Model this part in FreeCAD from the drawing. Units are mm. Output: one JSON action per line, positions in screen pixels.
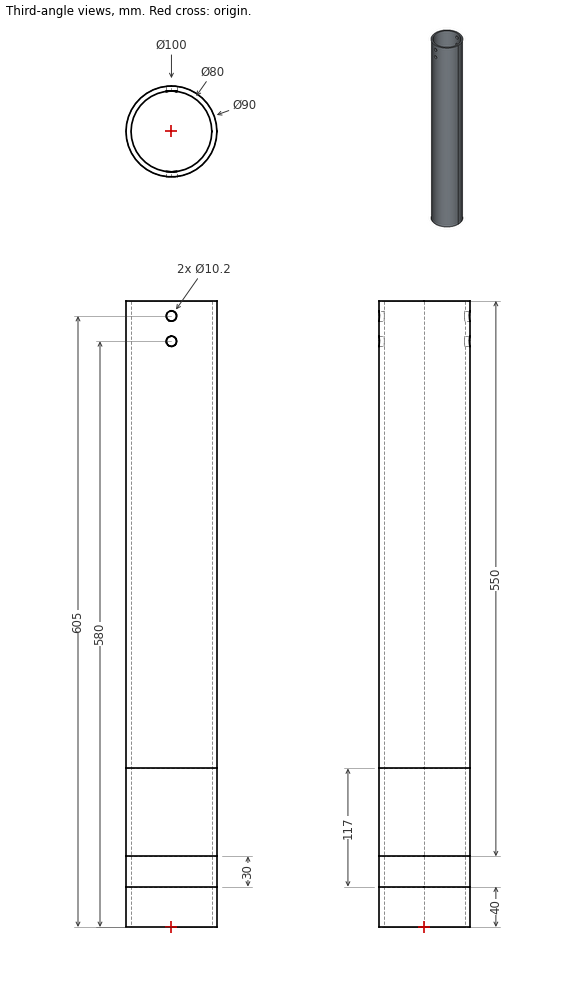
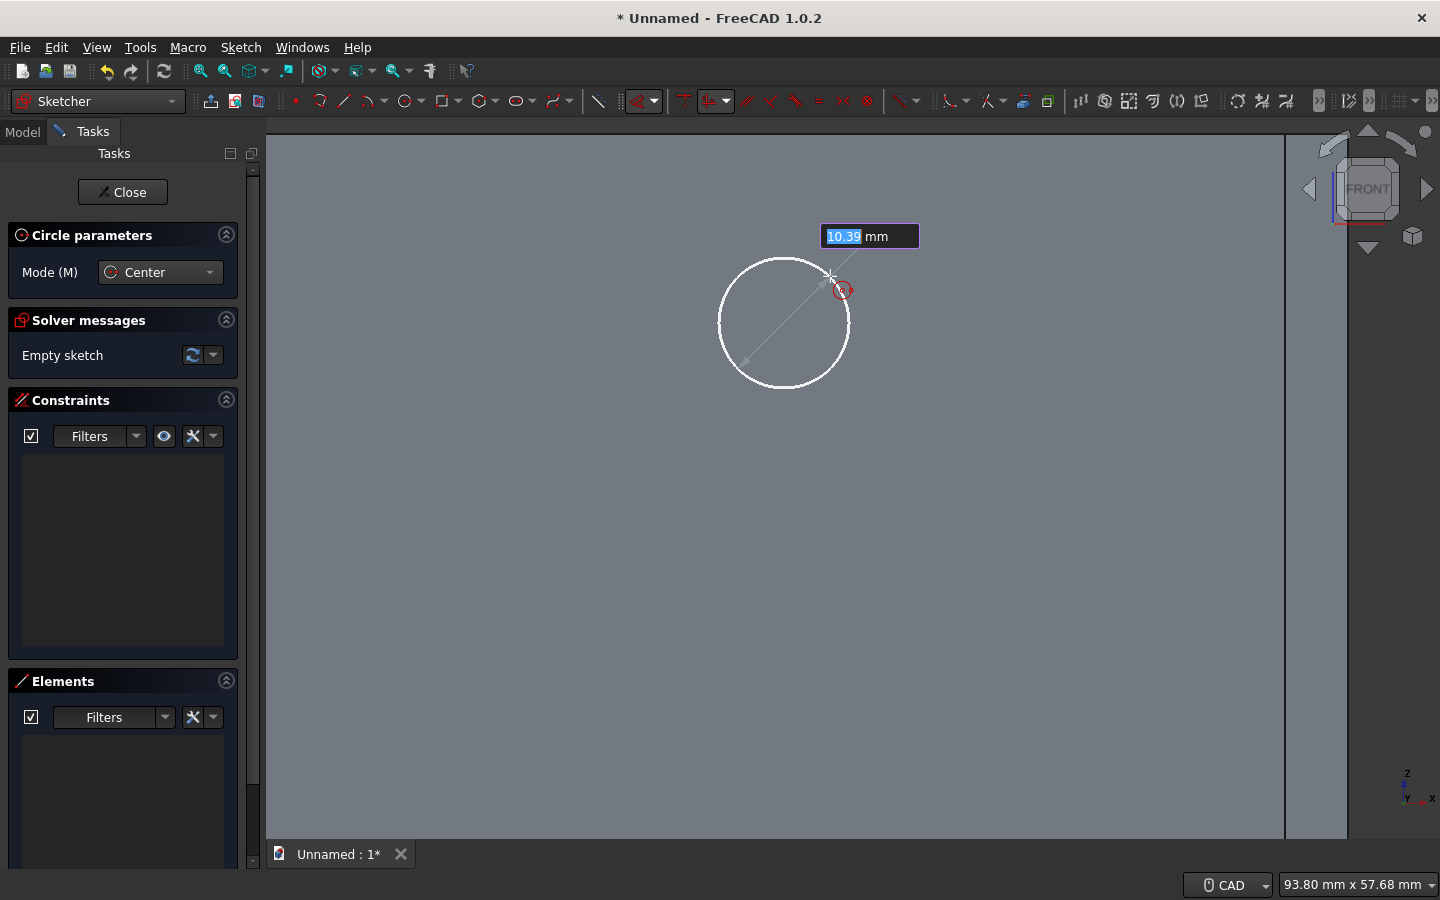
{"action": "type", "text": "10.2"}
{"action": "key", "text": "Return"}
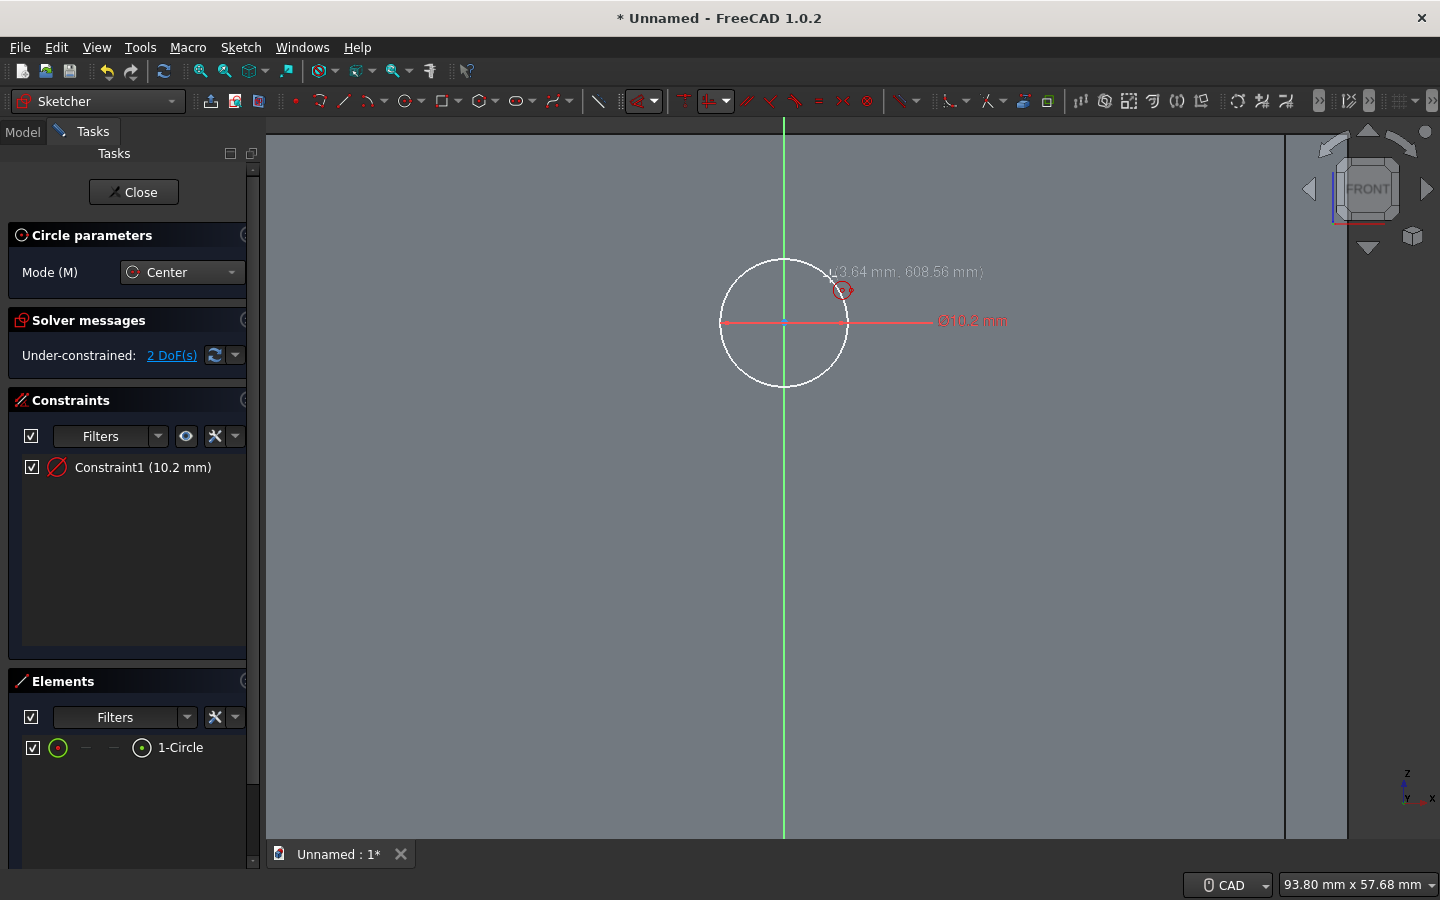
{"action": "left_click", "coordinate": [784, 634]}
{"action": "mouse_move", "coordinate": [830, 589]}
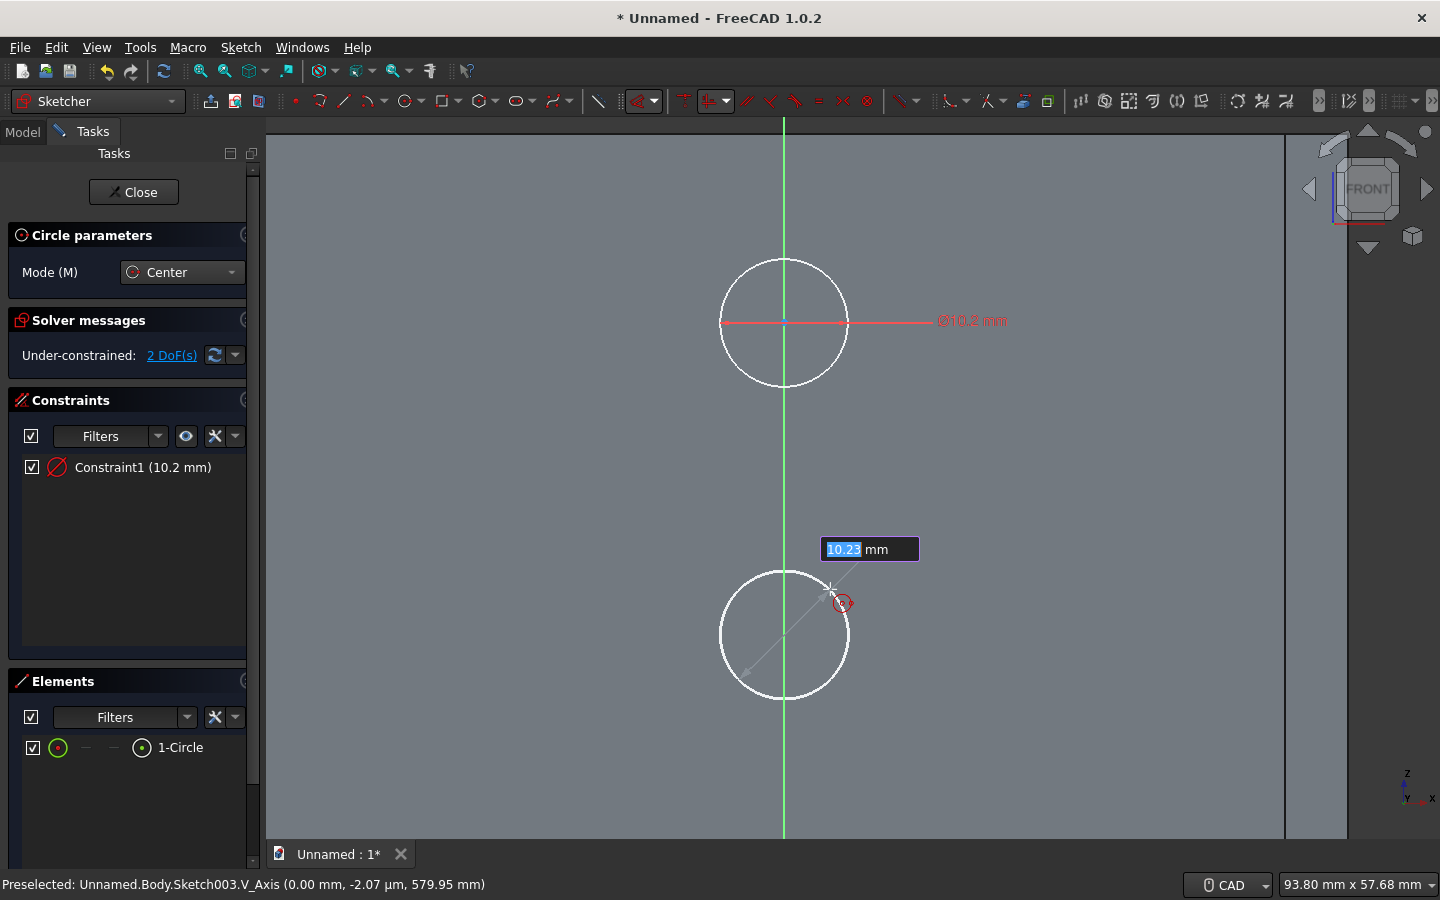
{"action": "type", "text": "10.2"}
{"action": "key", "text": "Return"}
{"action": "key", "text": "Escape"}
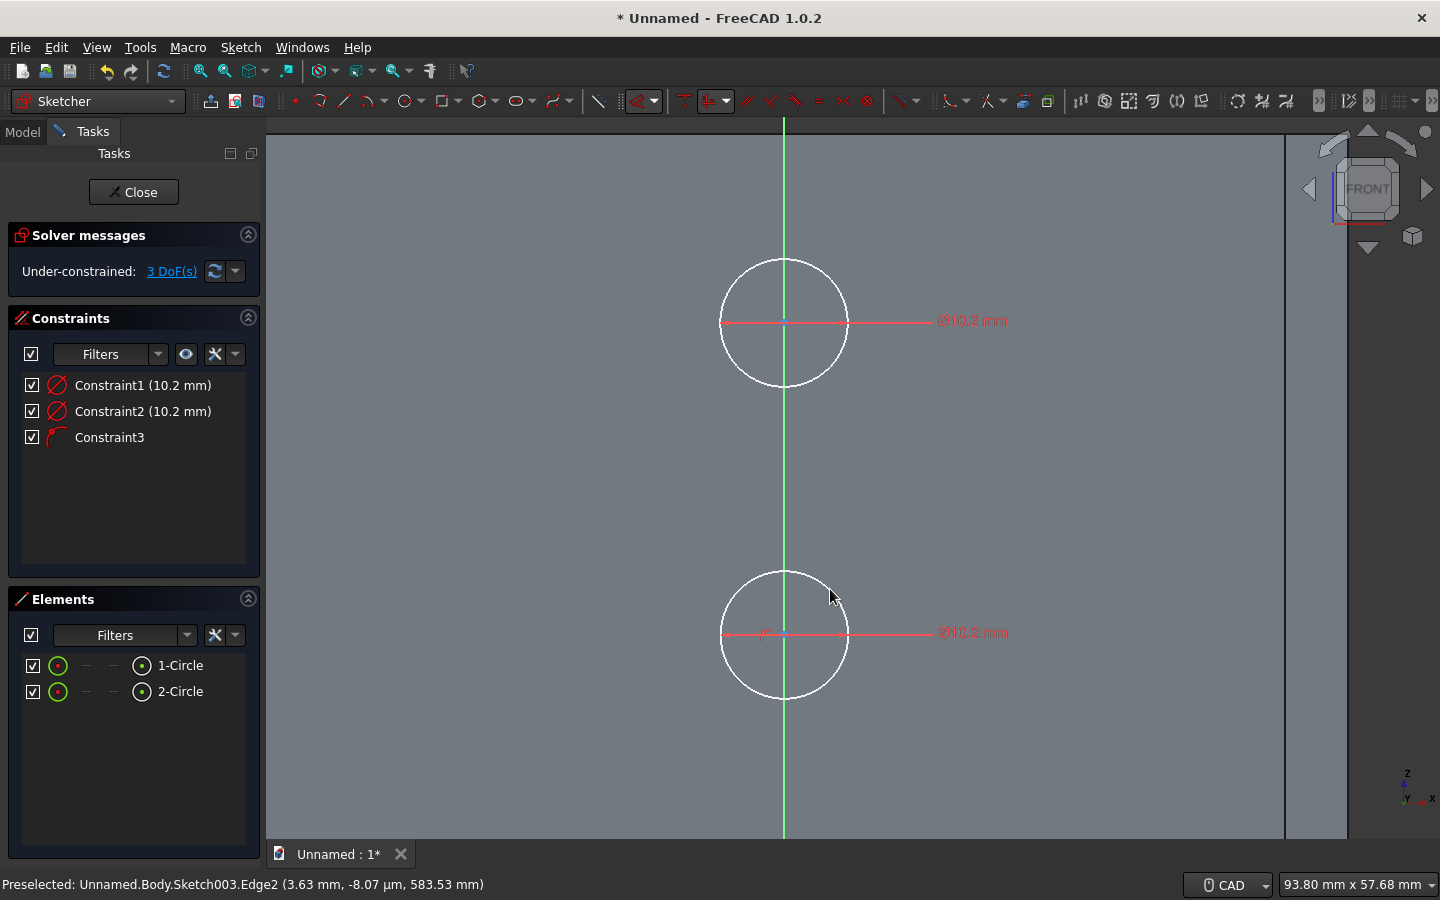
{"action": "left_click", "coordinate": [784, 323]}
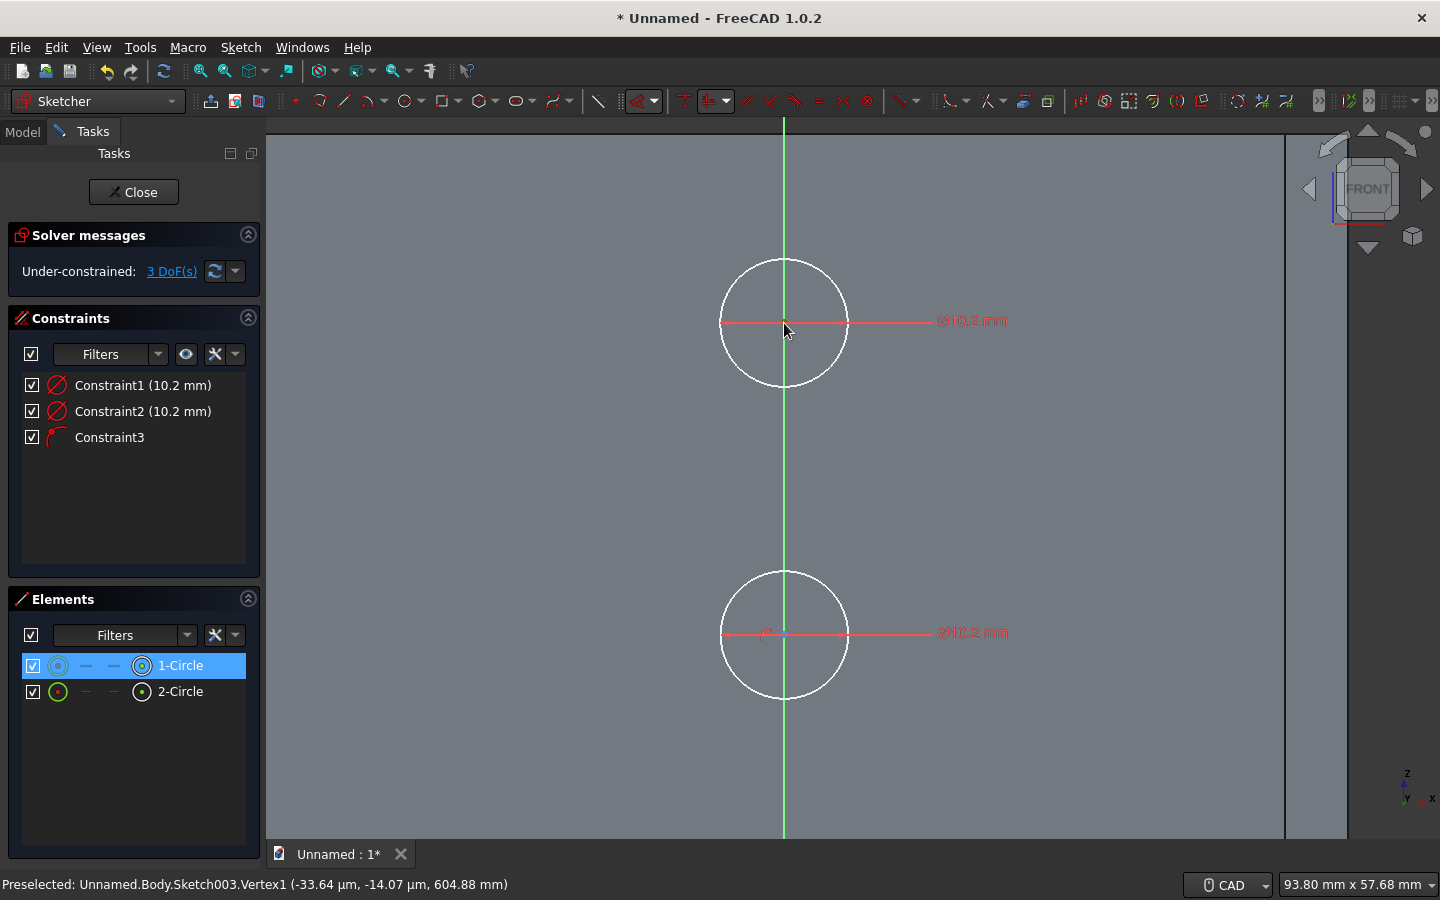
{"action": "left_click", "coordinate": [784, 763]}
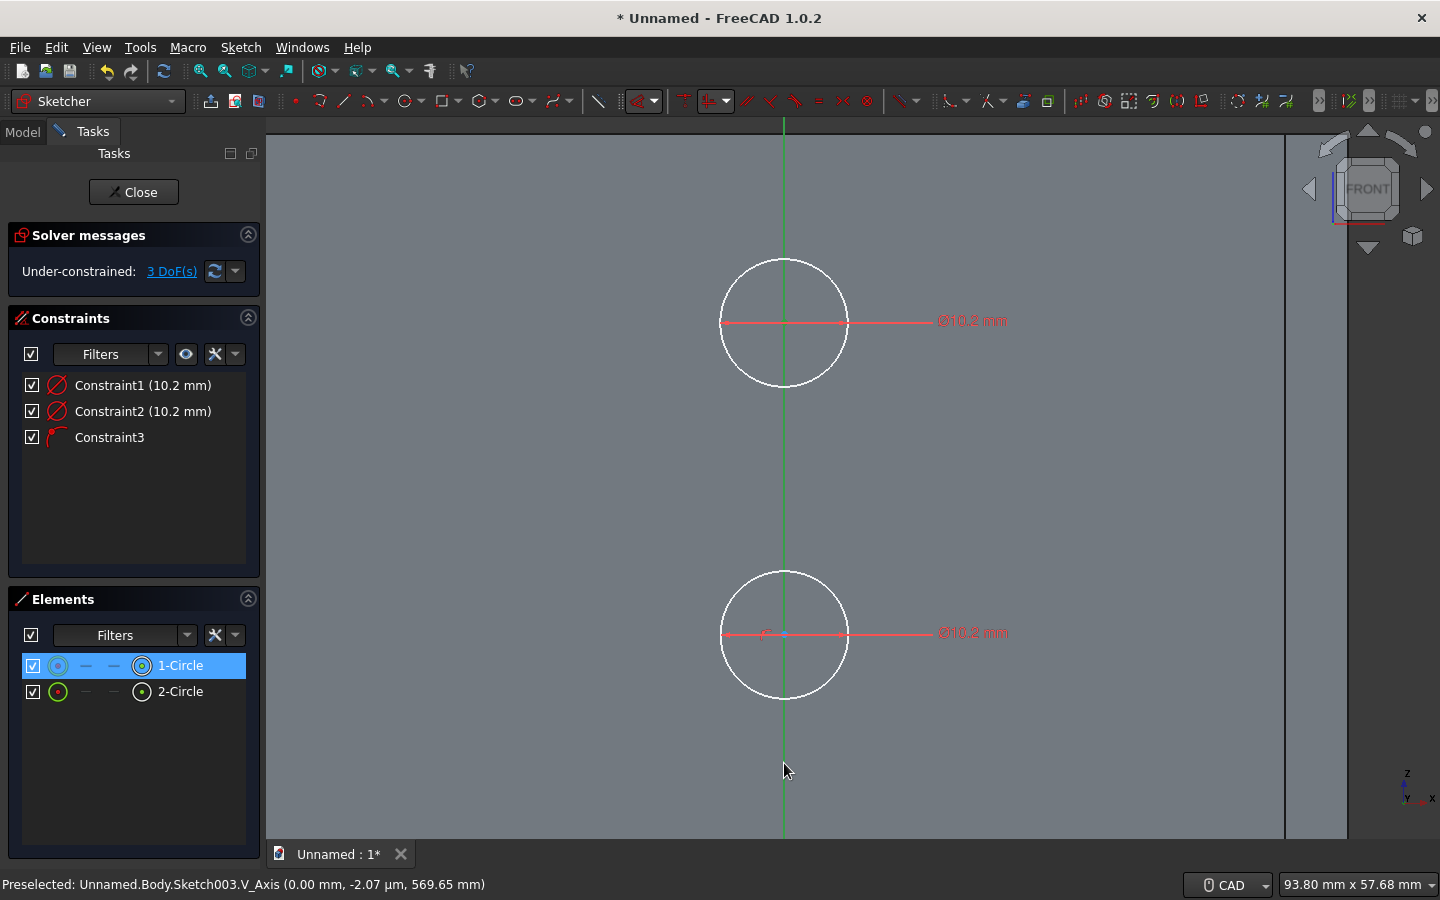
{"action": "key", "text": "c"}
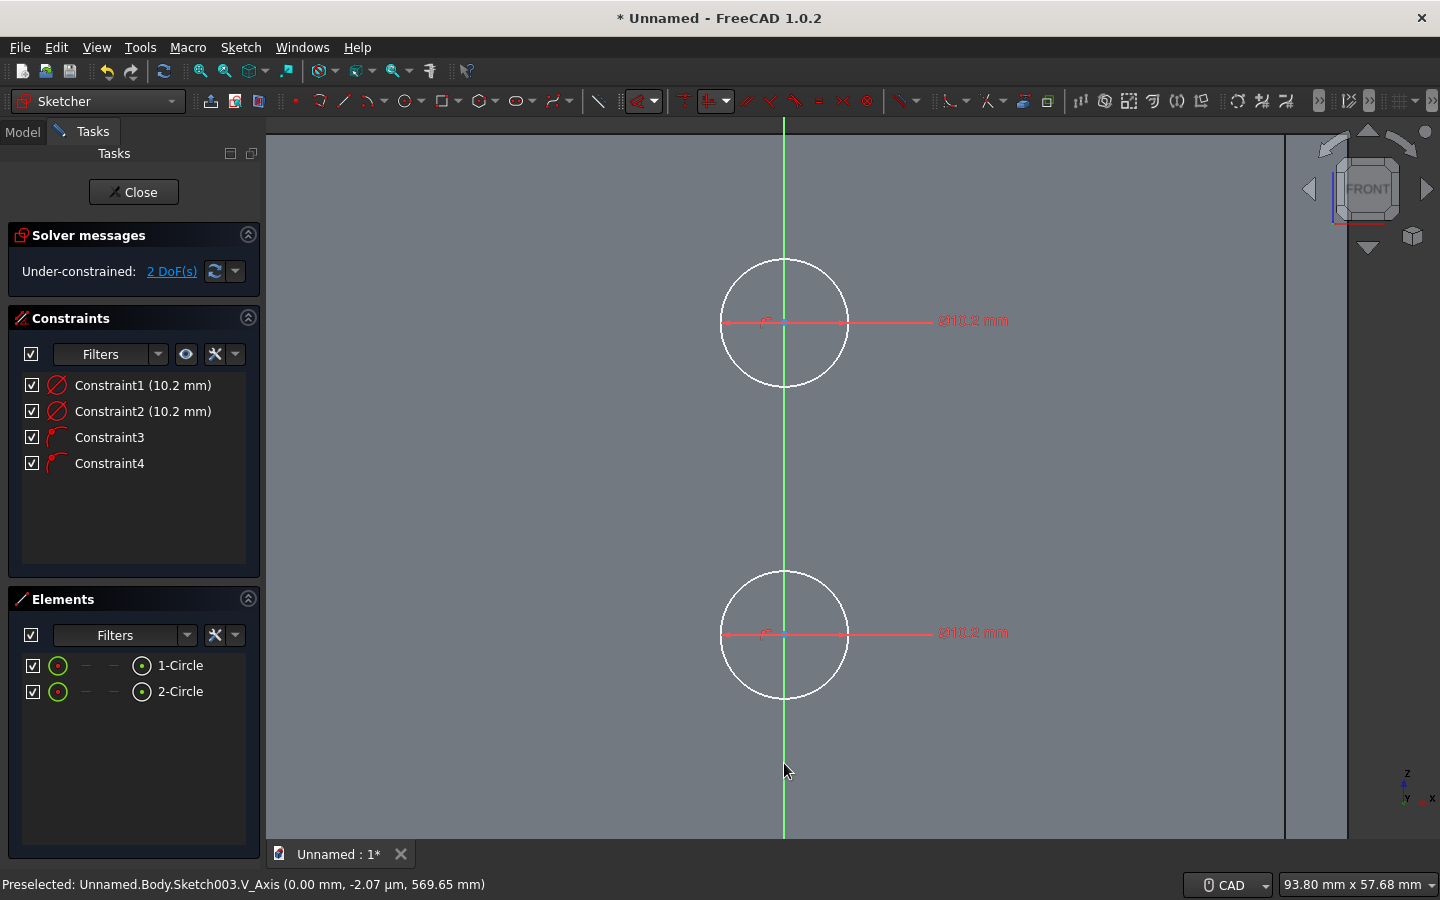
{"action": "left_click", "coordinate": [638, 102]}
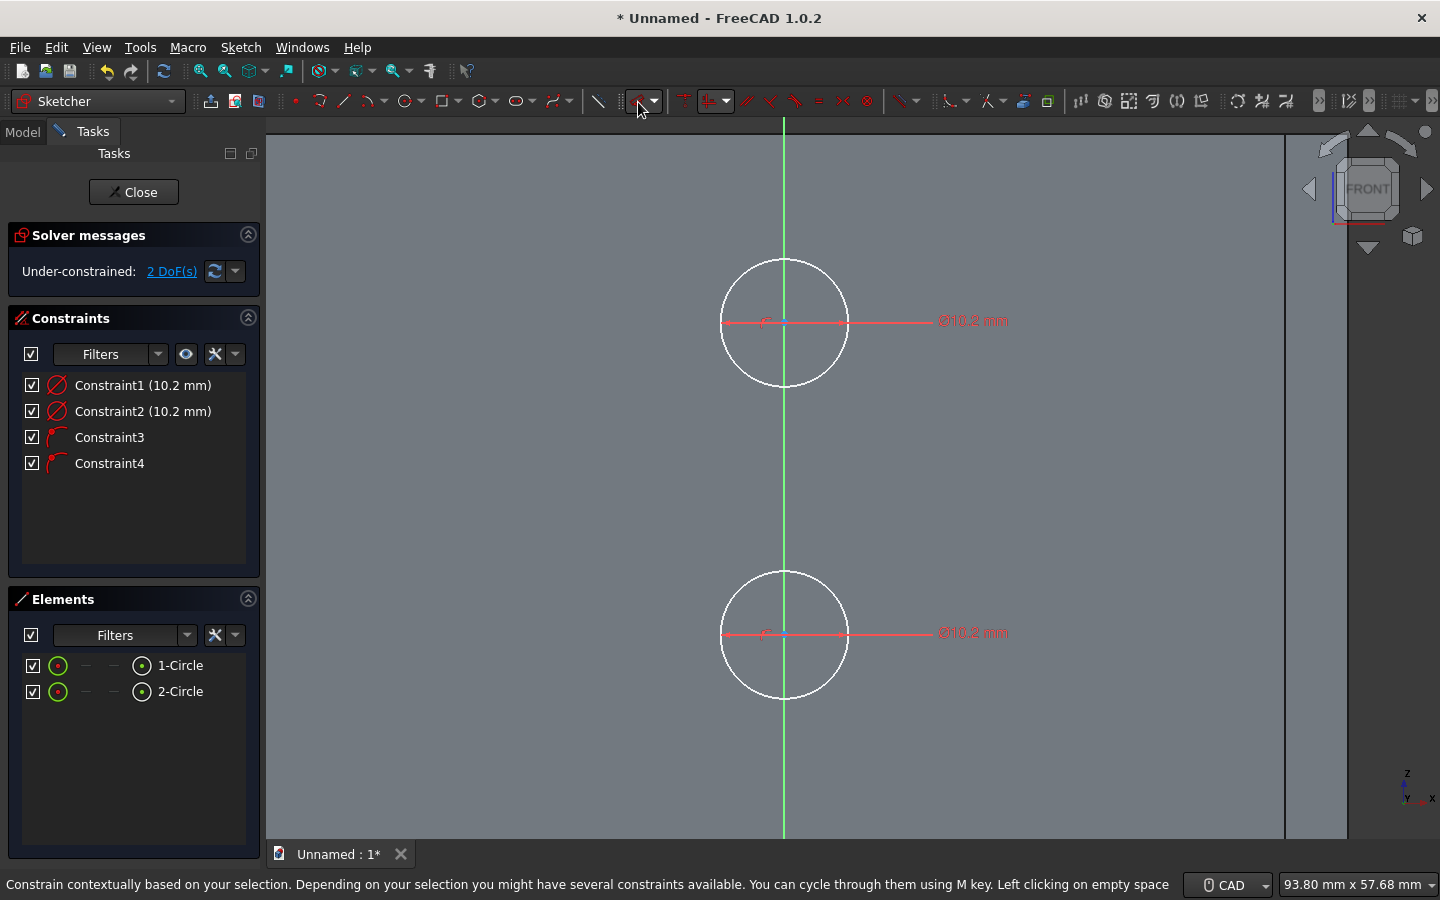
{"action": "left_click", "coordinate": [784, 323]}
{"action": "left_click", "coordinate": [818, 455]}